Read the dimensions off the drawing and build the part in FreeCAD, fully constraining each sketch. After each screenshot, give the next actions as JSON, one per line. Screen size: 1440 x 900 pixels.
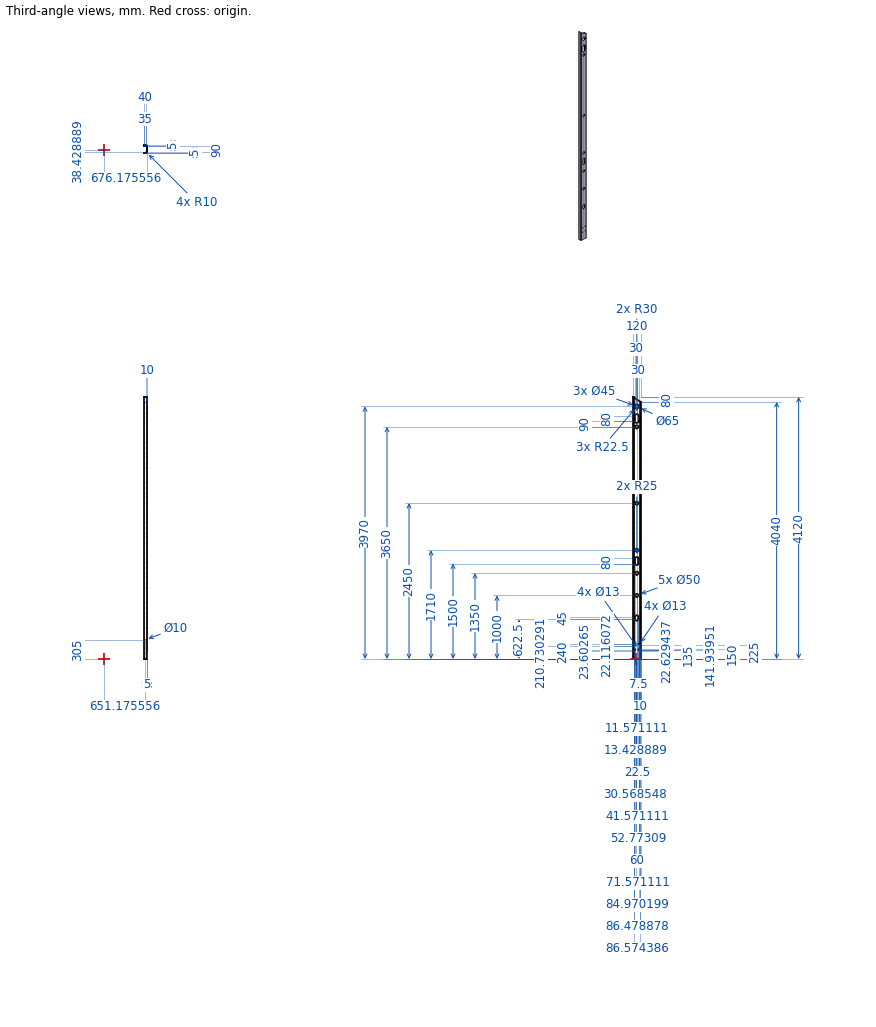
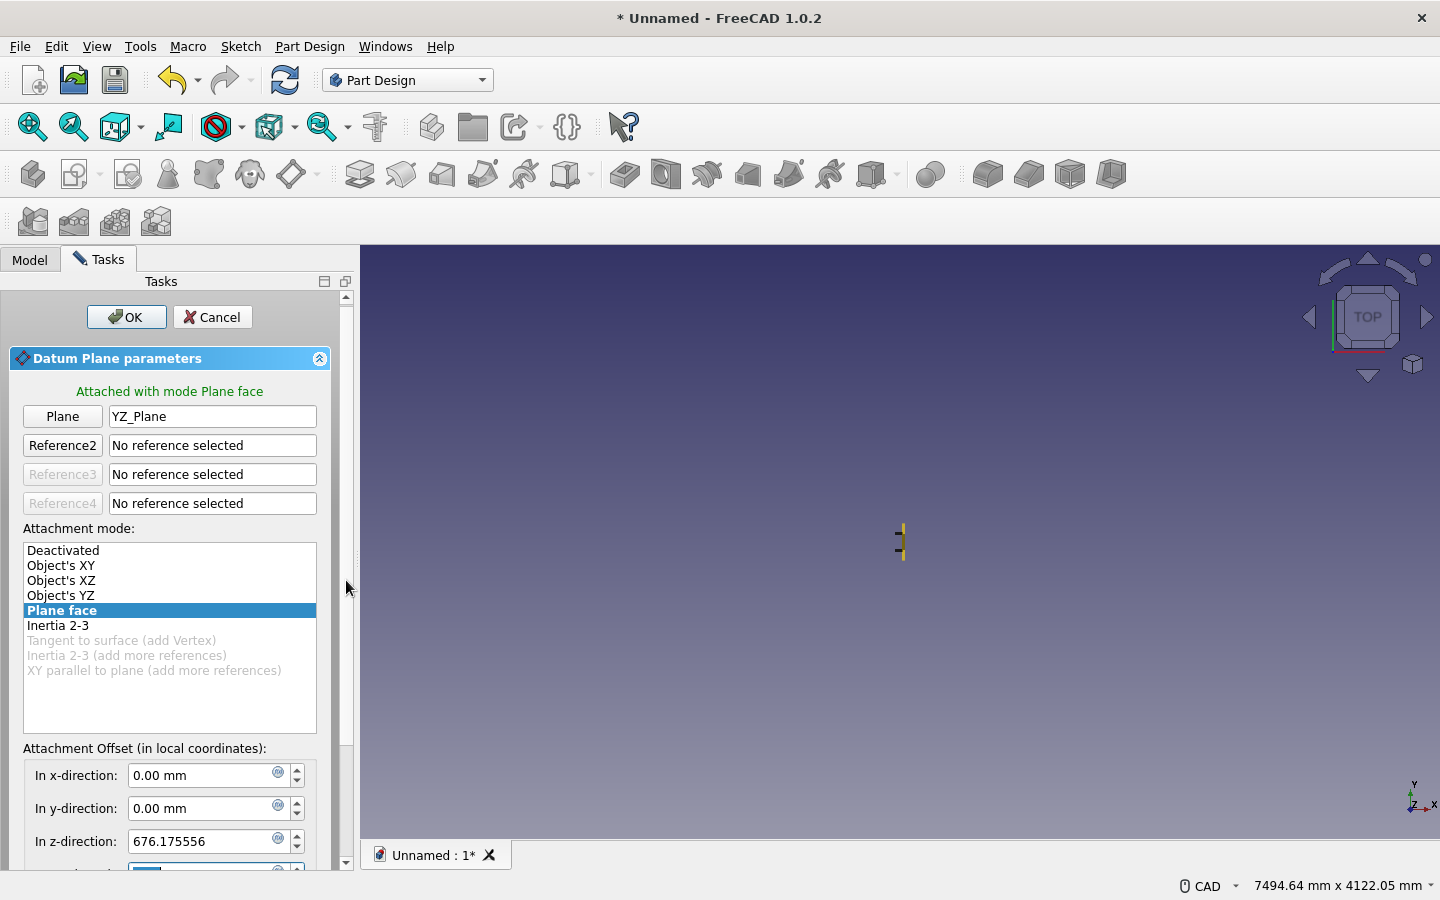
{"action": "left_click", "coordinate": [127, 320]}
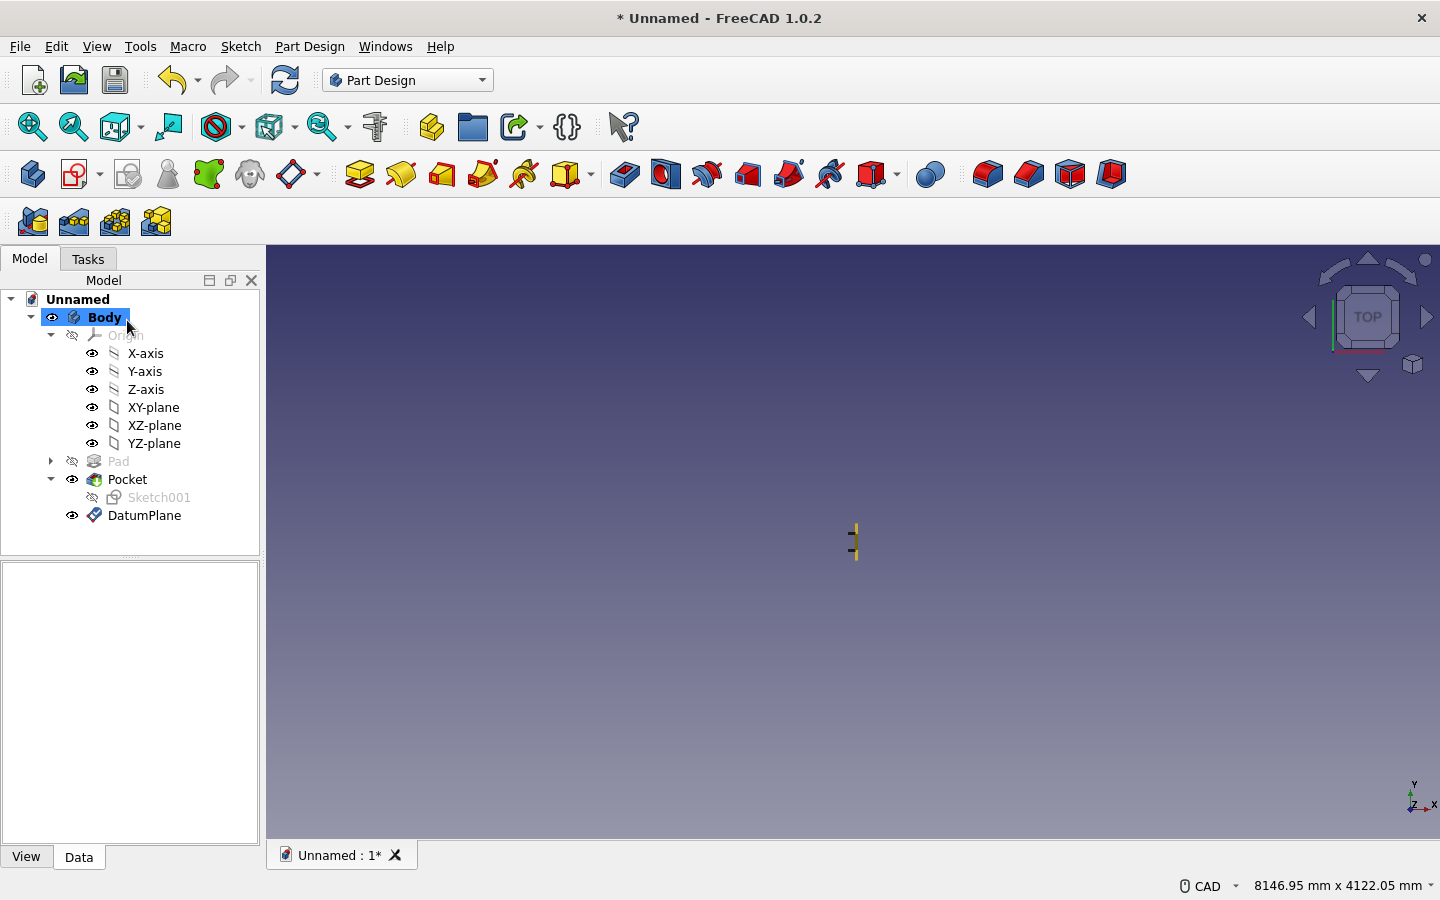
{"action": "left_click", "coordinate": [117, 515]}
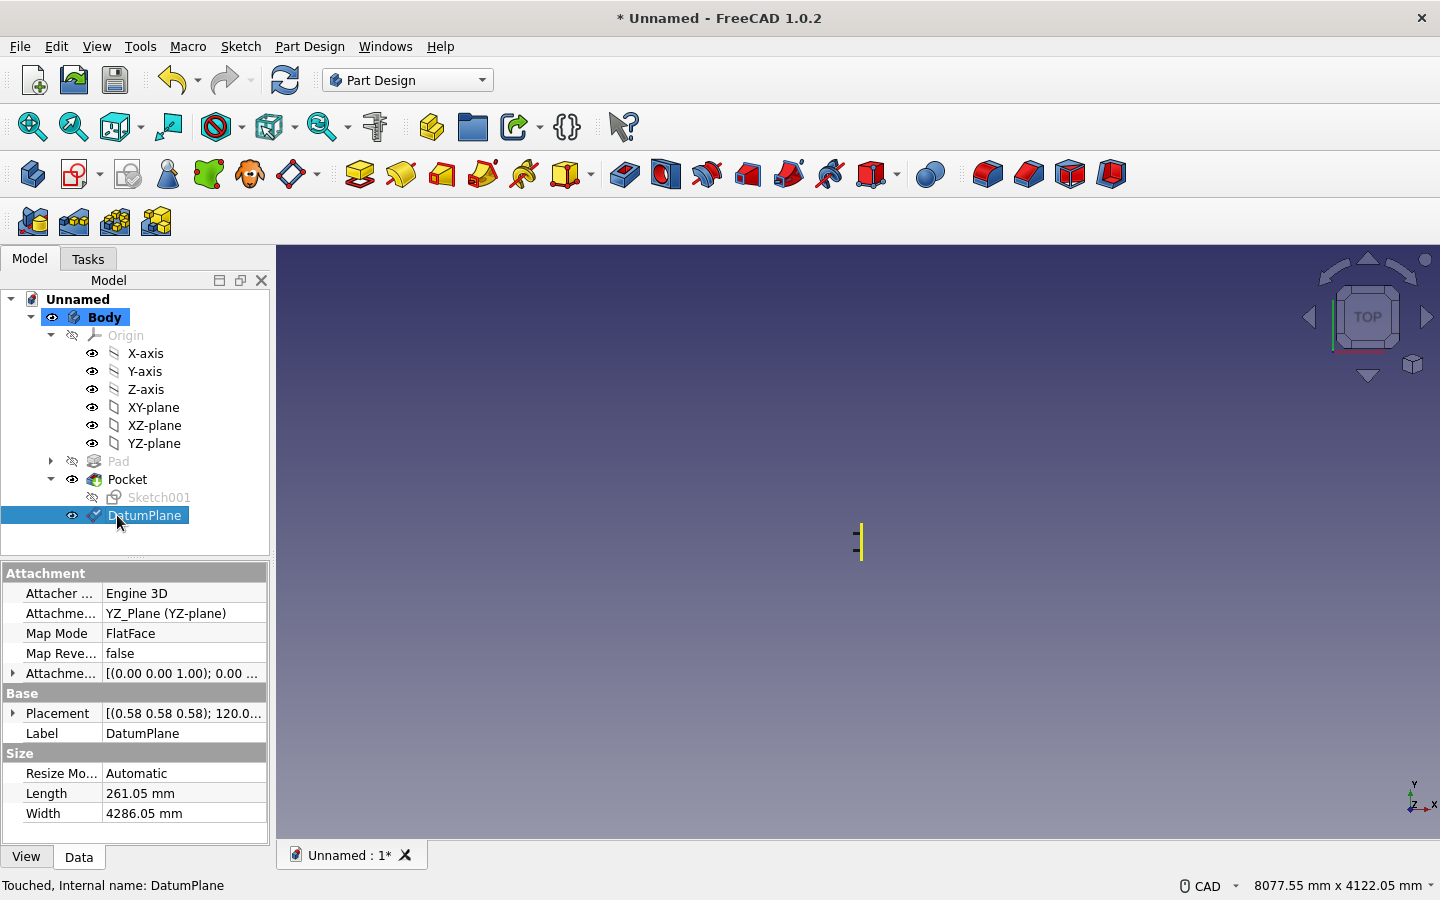
{"action": "left_click", "coordinate": [74, 174]}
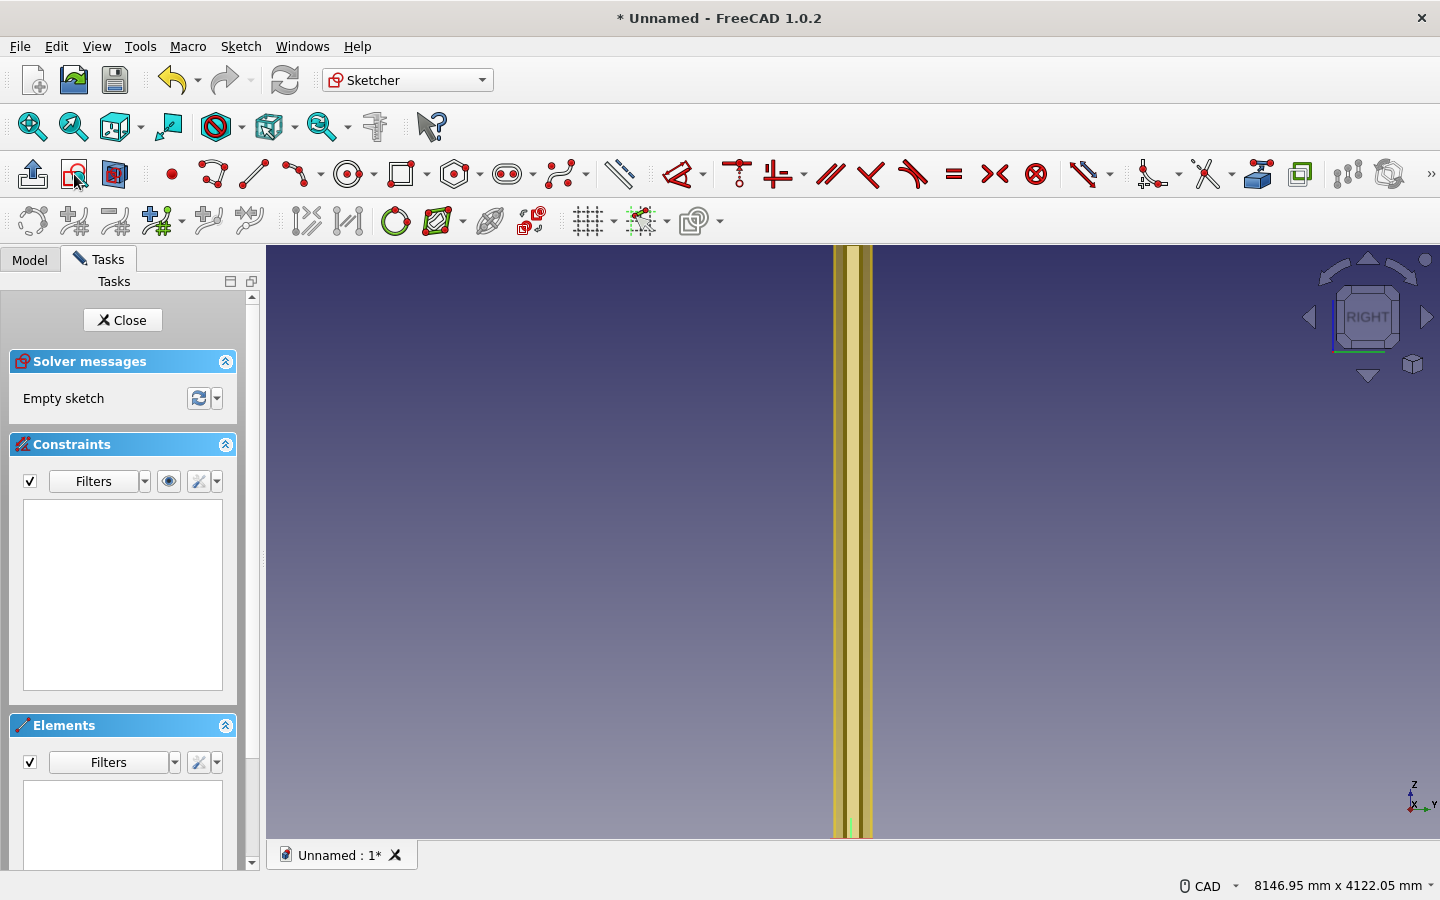
{"action": "scroll", "coordinate": [645, 523], "scroll_direction": "down", "scroll_amount": 2}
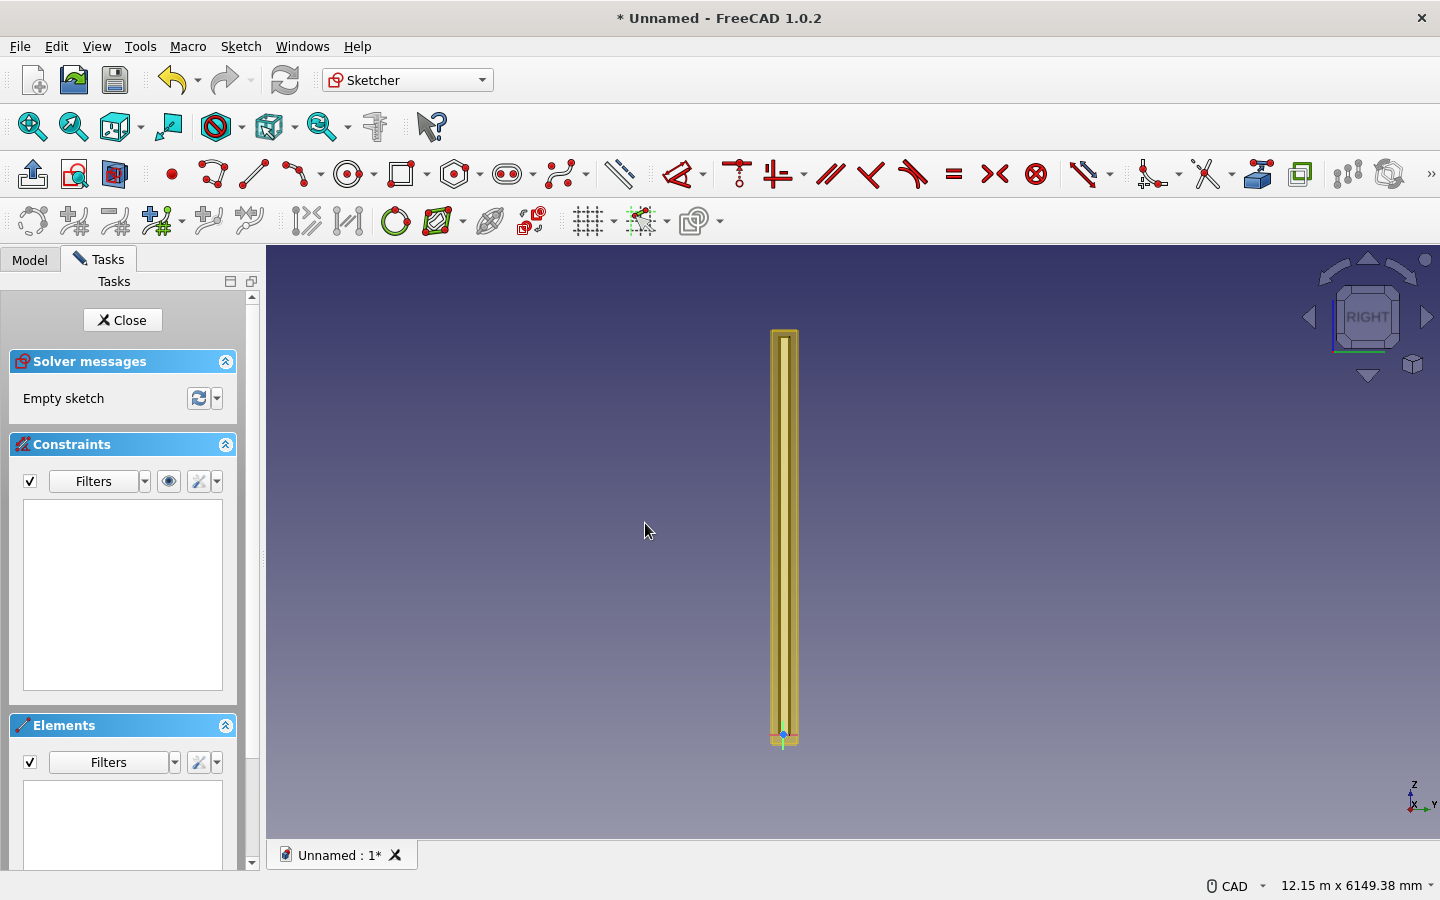
{"action": "left_click", "coordinate": [506, 174]}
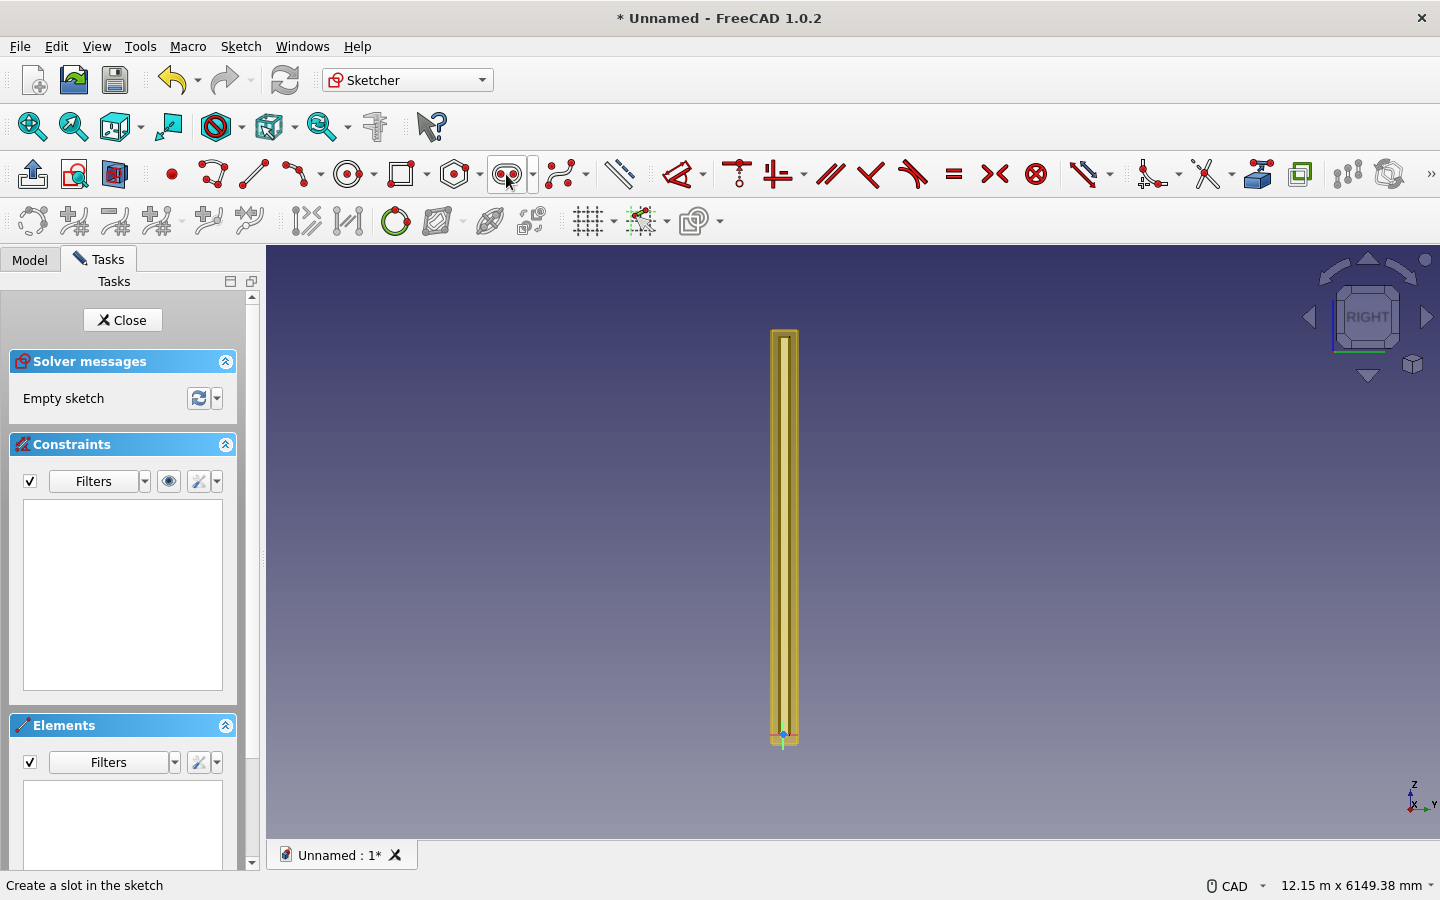
{"action": "scroll", "coordinate": [785, 675], "scroll_direction": "up", "scroll_amount": 14}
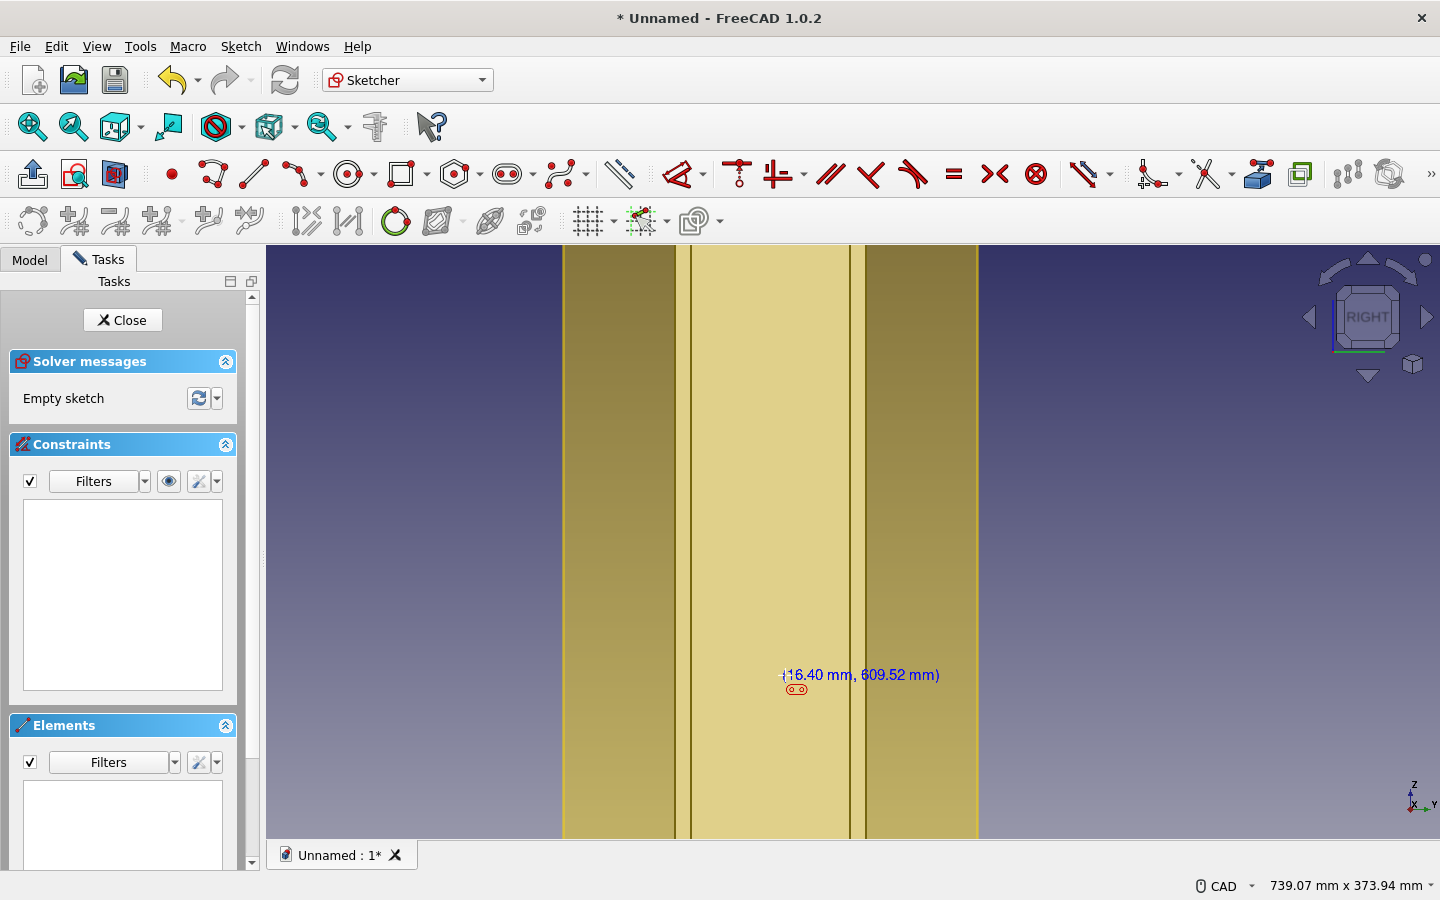
{"action": "left_click", "coordinate": [770, 660]}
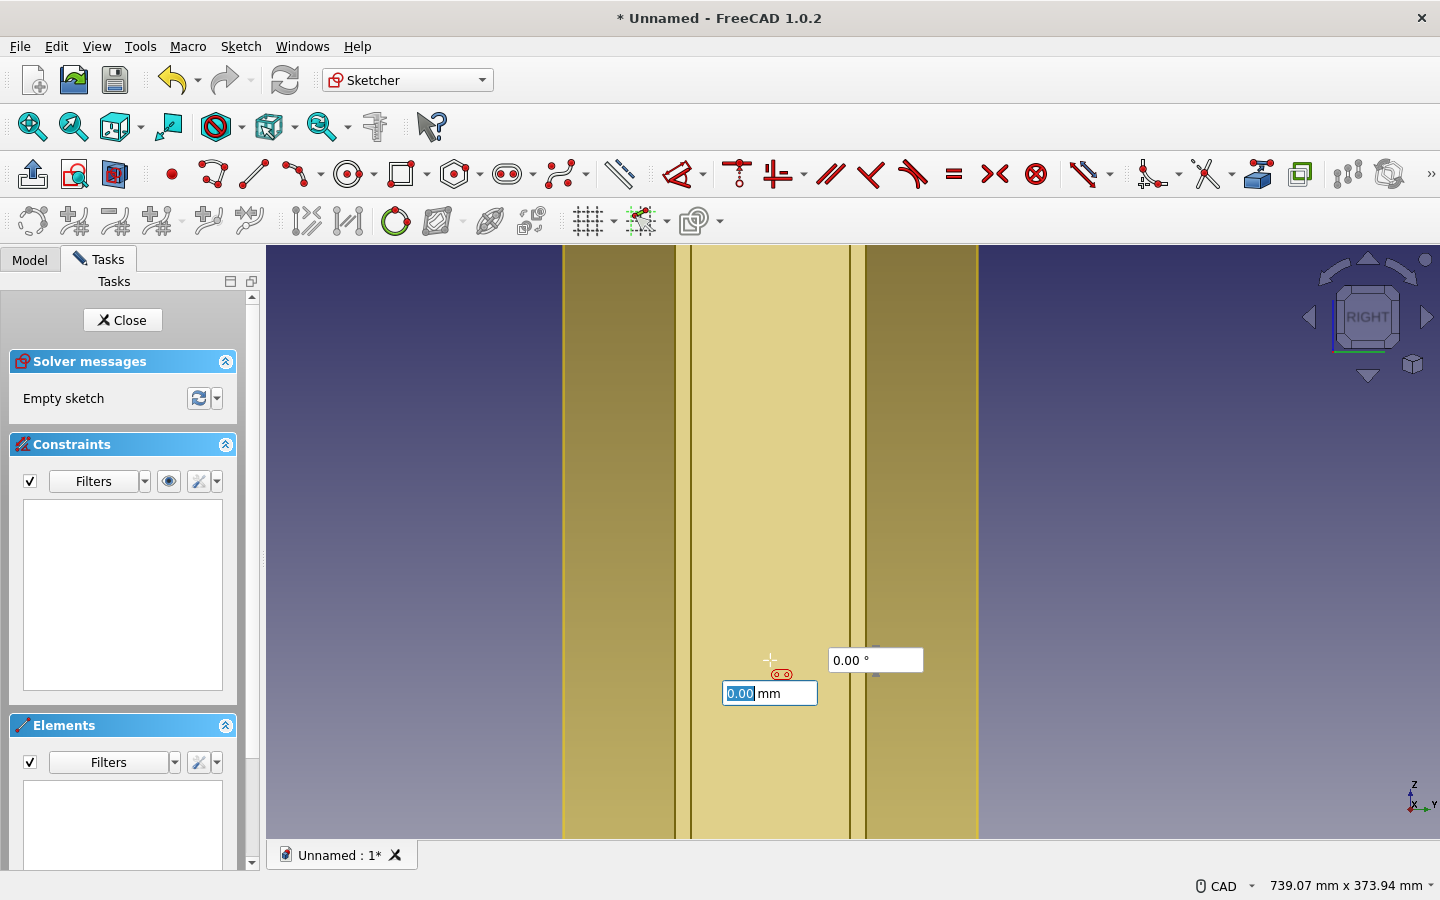
{"action": "left_click", "coordinate": [770, 588]}